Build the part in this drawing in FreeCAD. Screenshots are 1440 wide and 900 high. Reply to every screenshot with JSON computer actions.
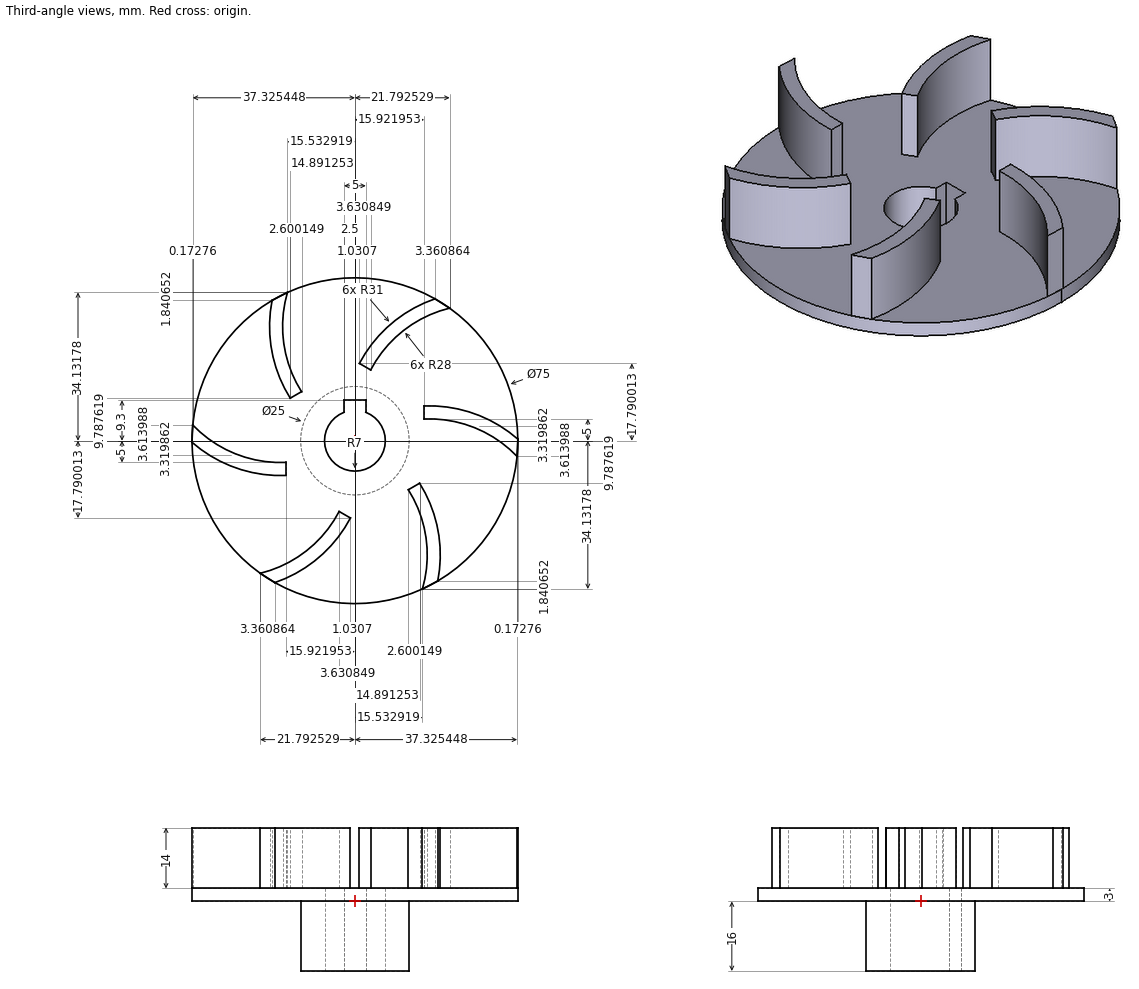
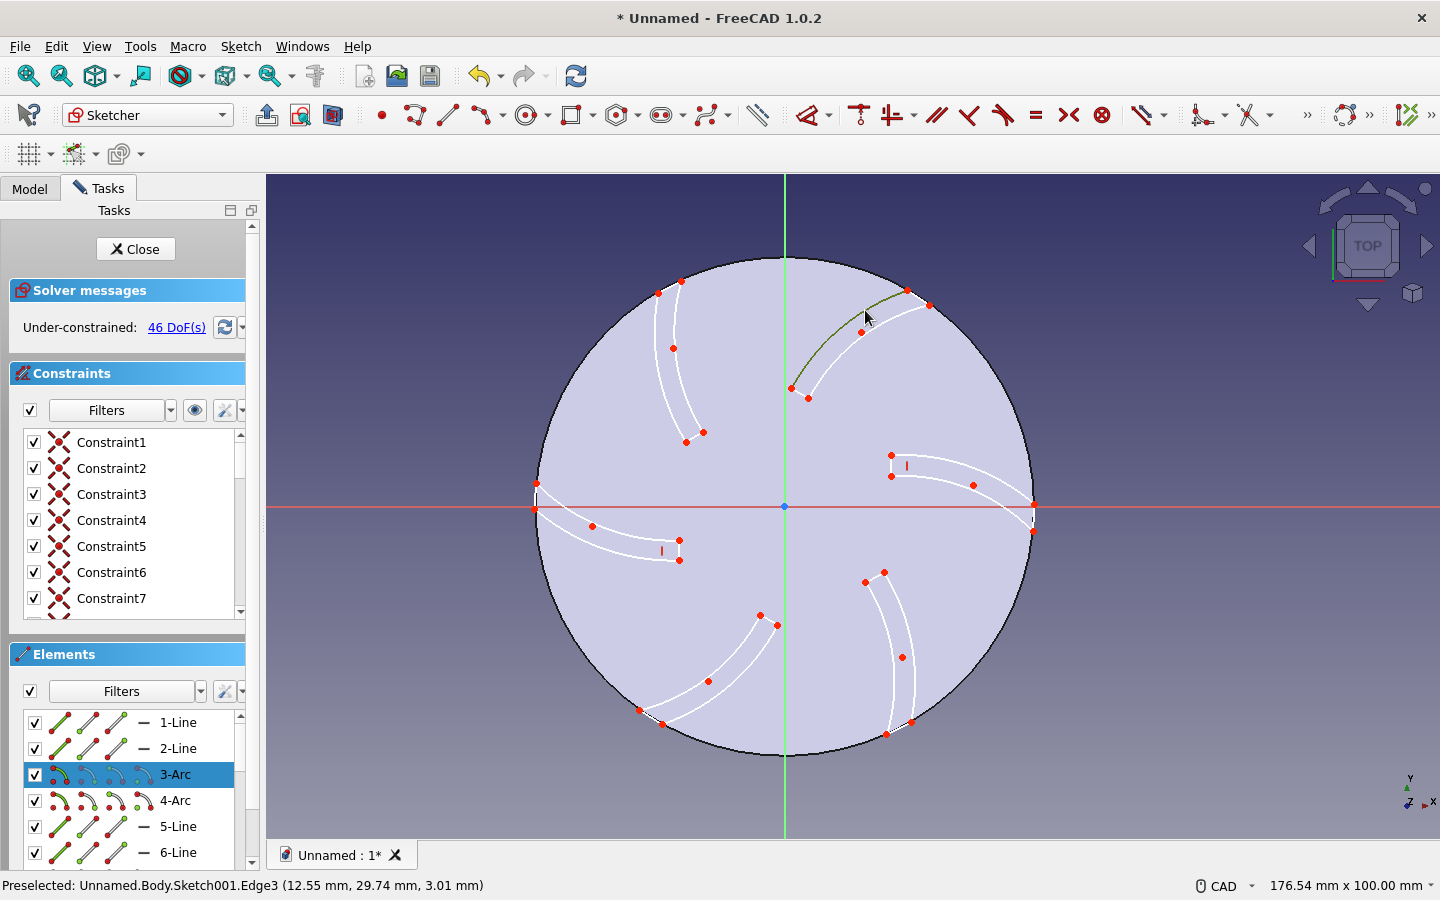
{"action": "left_click", "coordinate": [655, 339]}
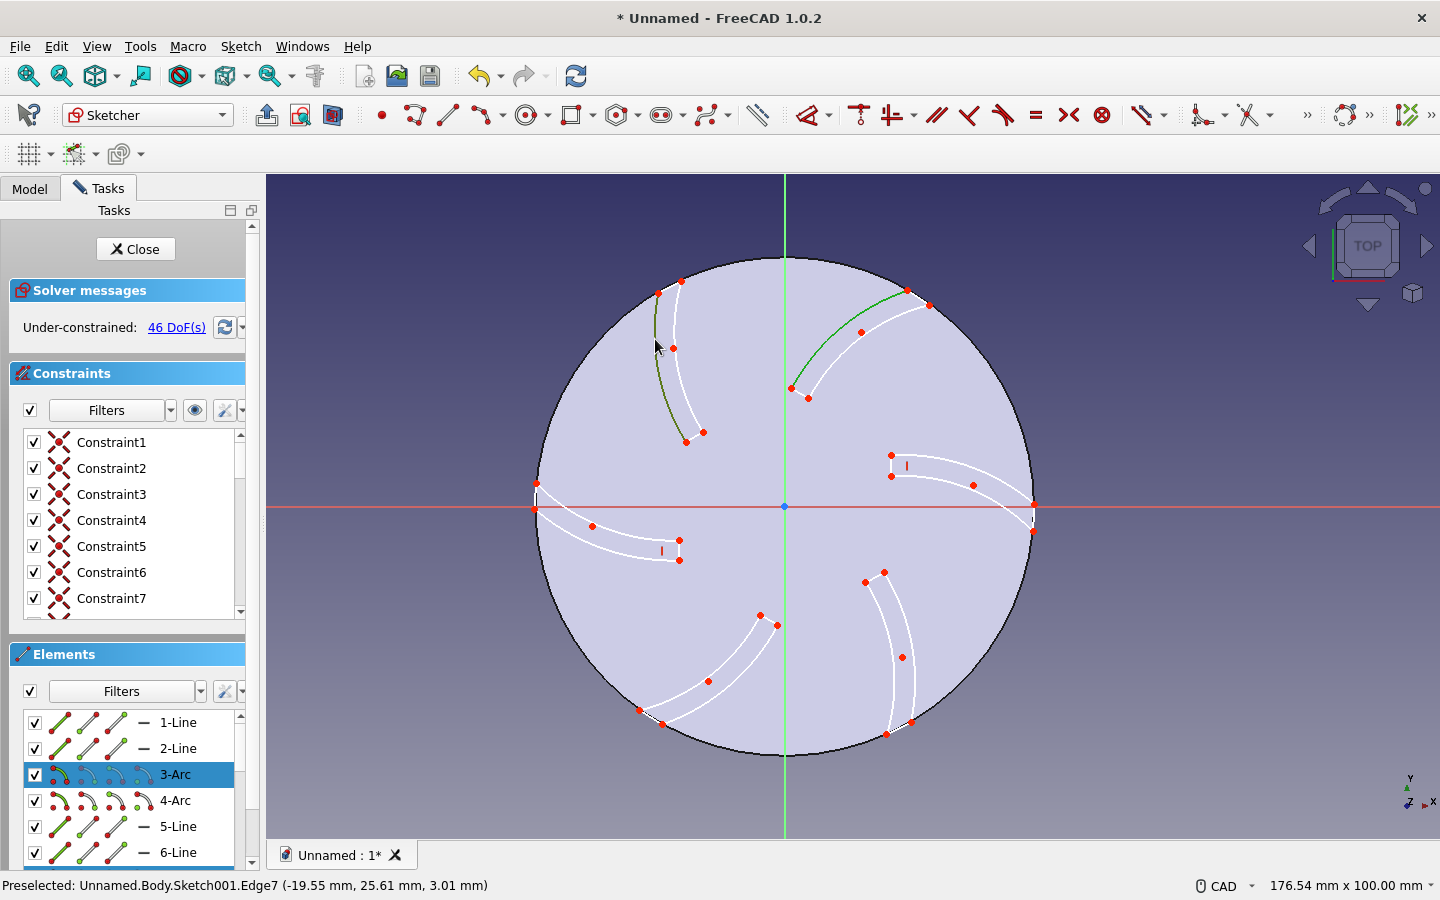
{"action": "left_click", "coordinate": [573, 536]}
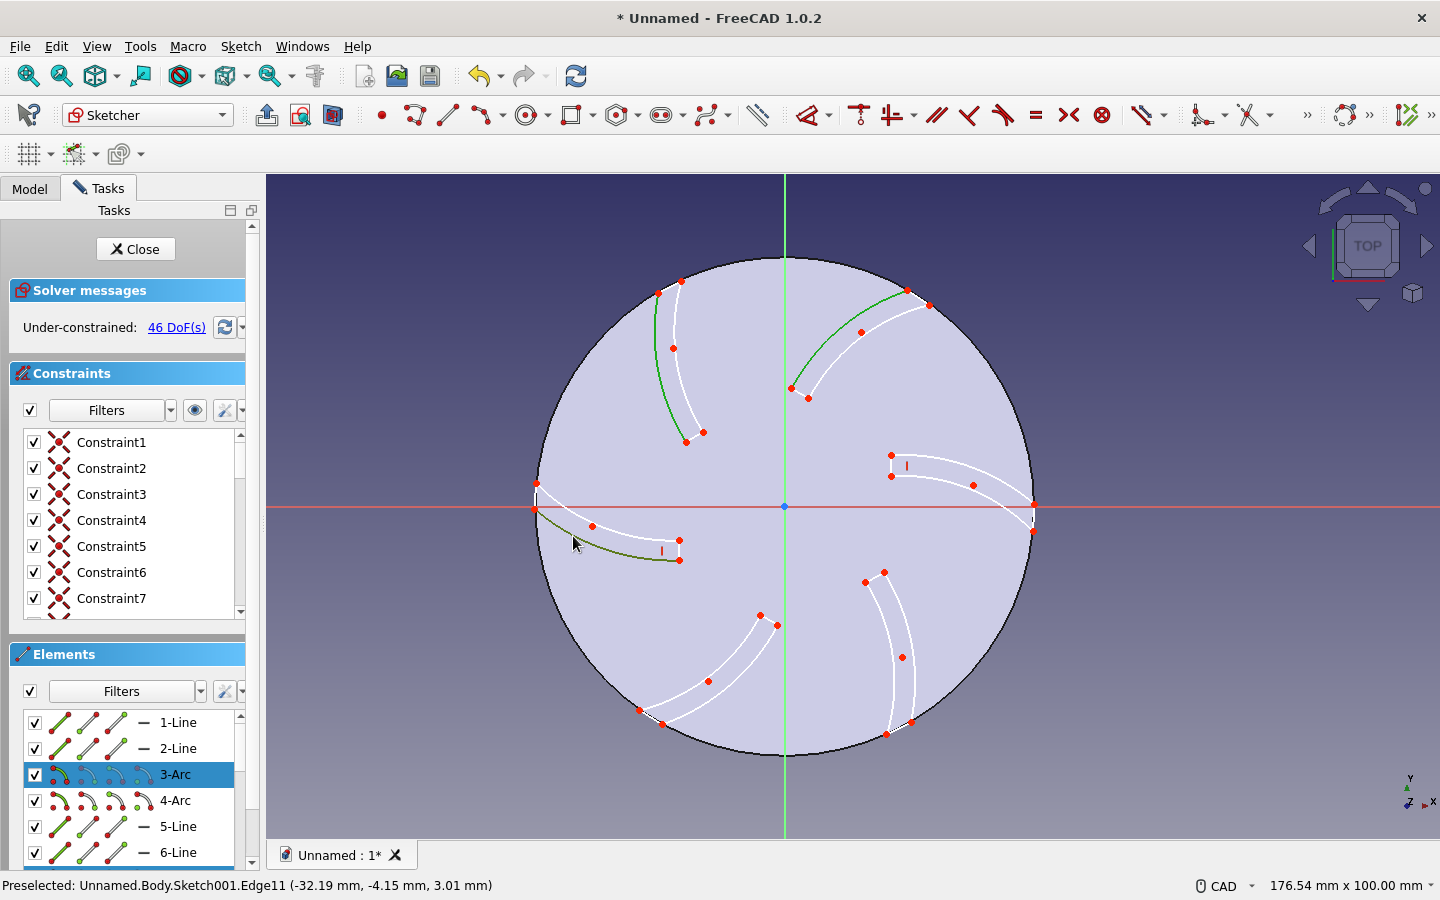
{"action": "left_click", "coordinate": [704, 704]}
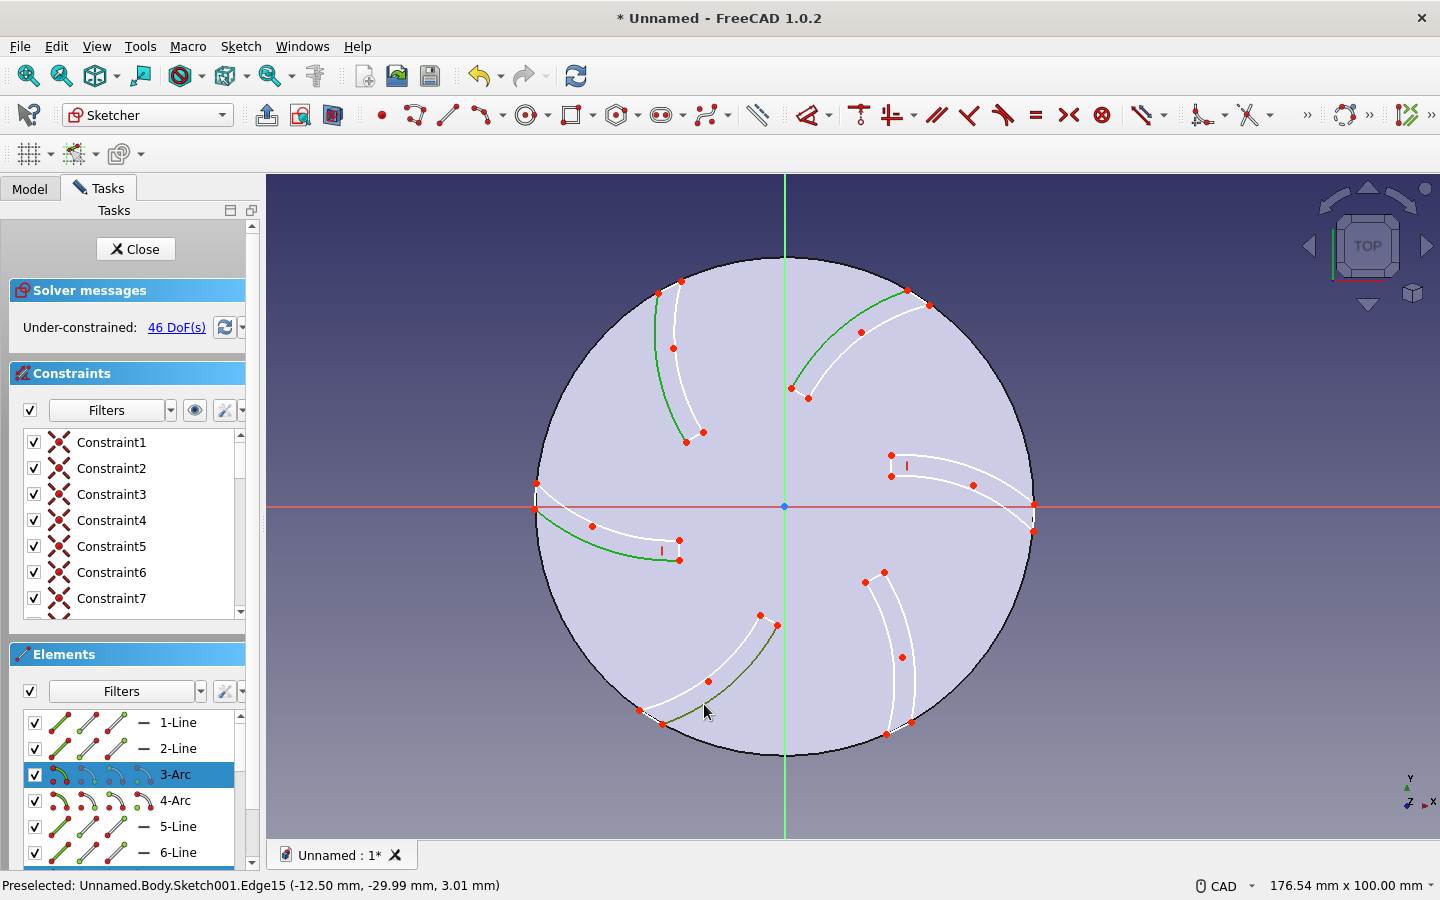
{"action": "left_click", "coordinate": [915, 676]}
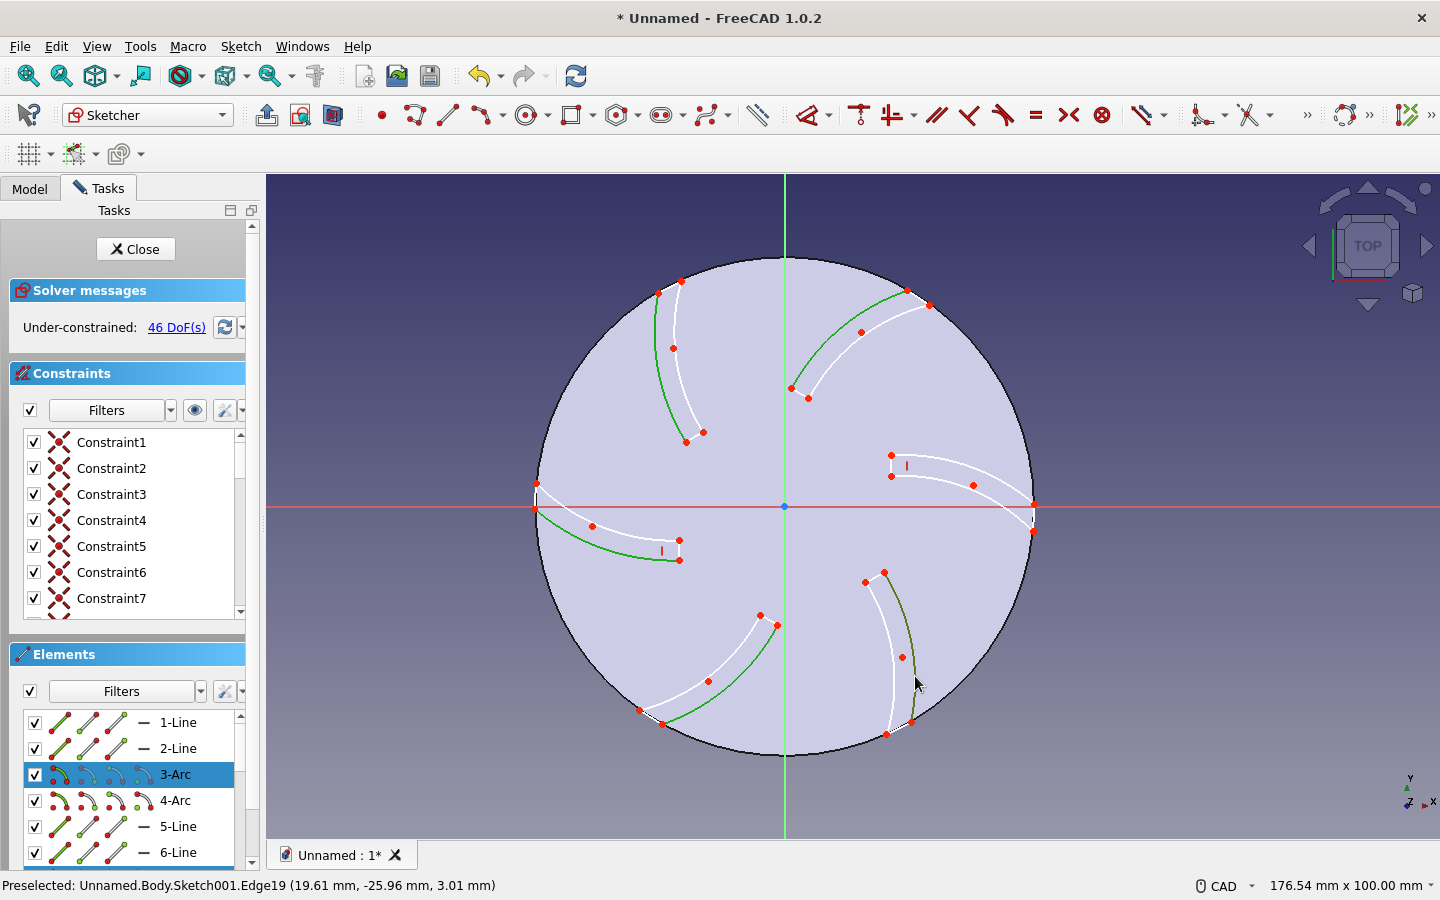
{"action": "left_click", "coordinate": [996, 478]}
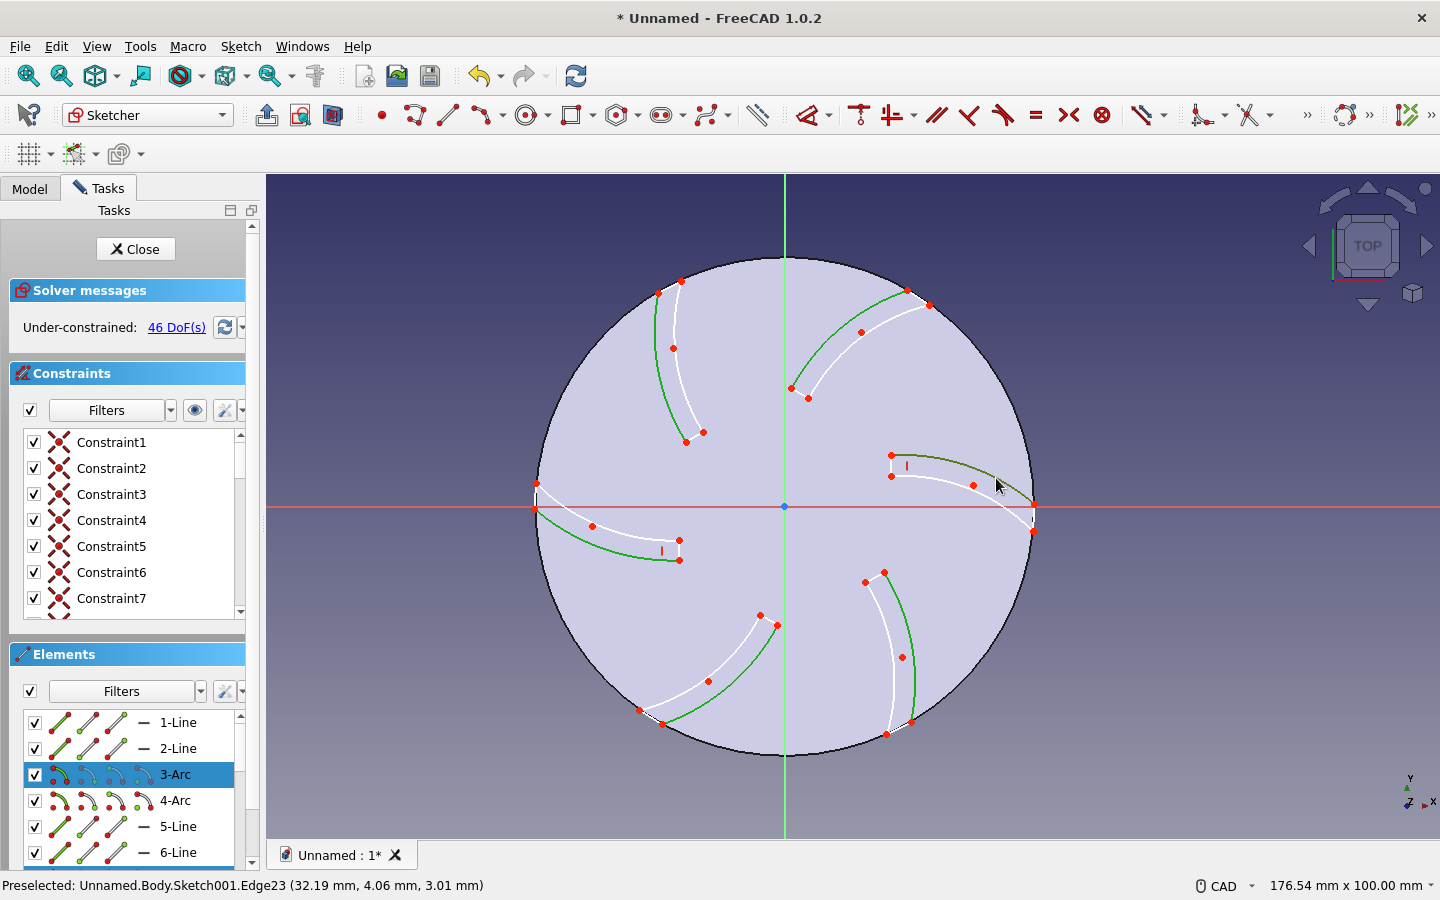
{"action": "key", "text": "e"}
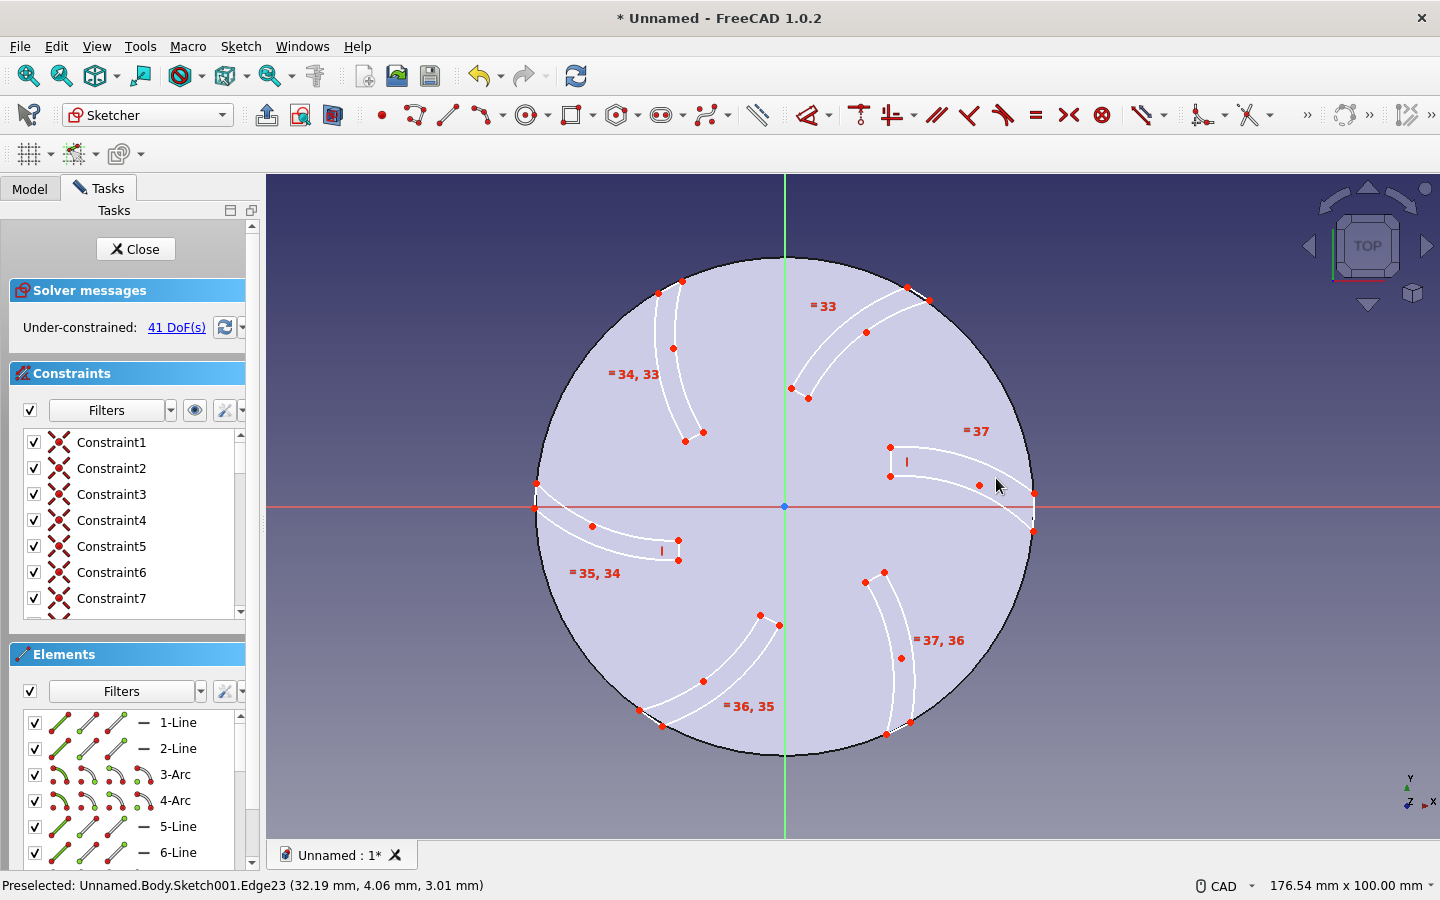
{"action": "left_click", "coordinate": [885, 319]}